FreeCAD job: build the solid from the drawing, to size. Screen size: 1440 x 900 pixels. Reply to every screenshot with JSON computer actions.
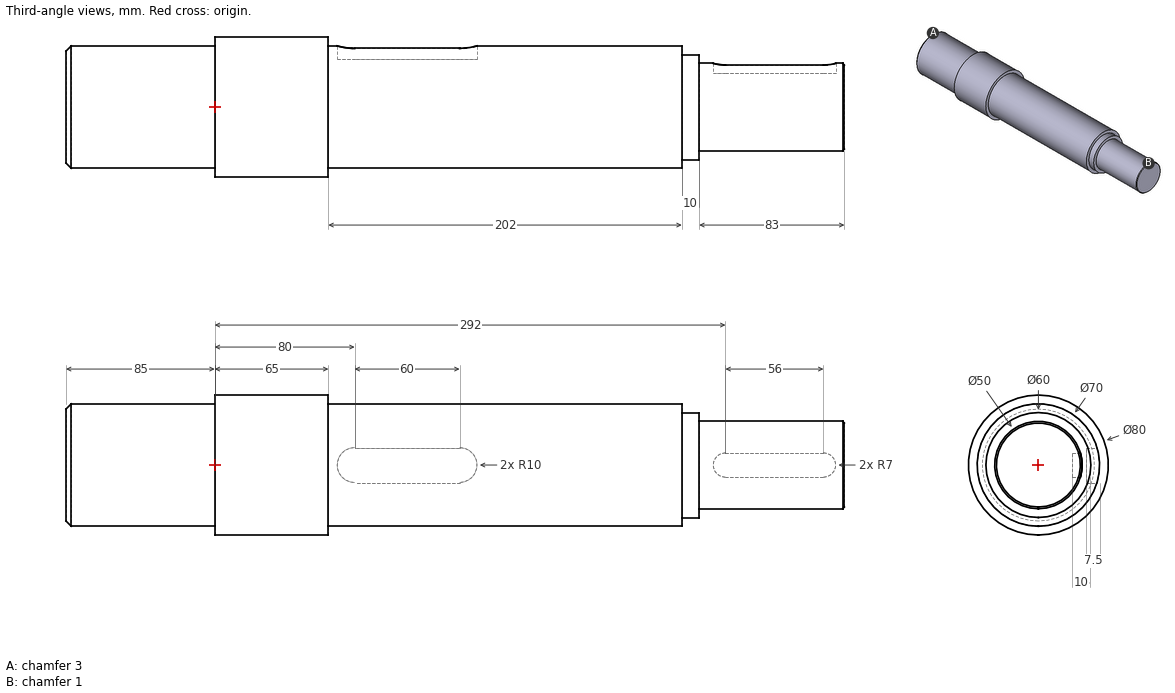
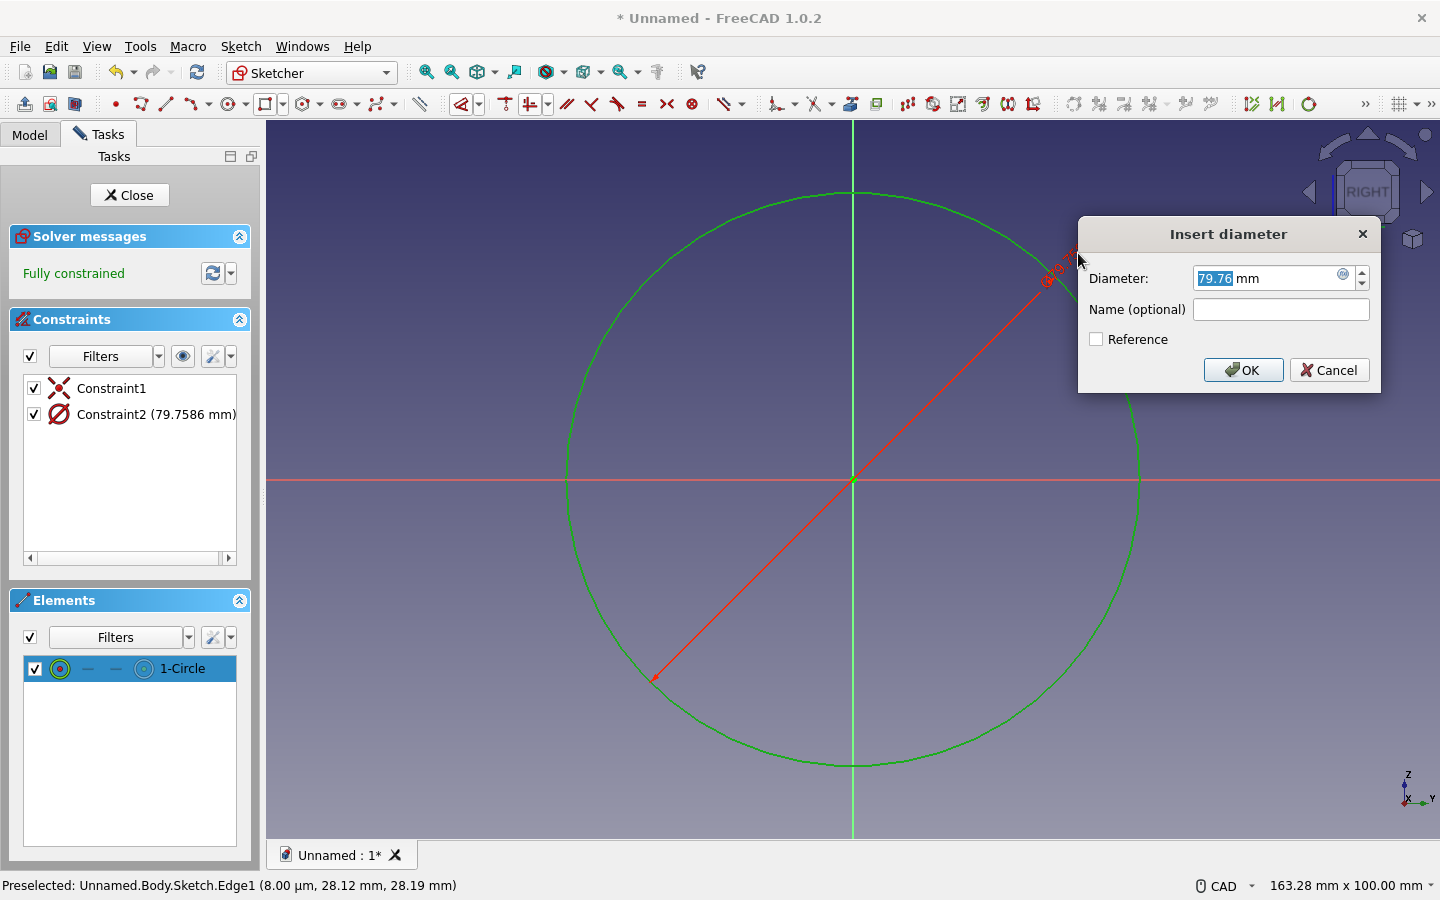
{"action": "type", "text": "80"}
{"action": "key", "text": "Return"}
{"action": "key", "text": "Escape"}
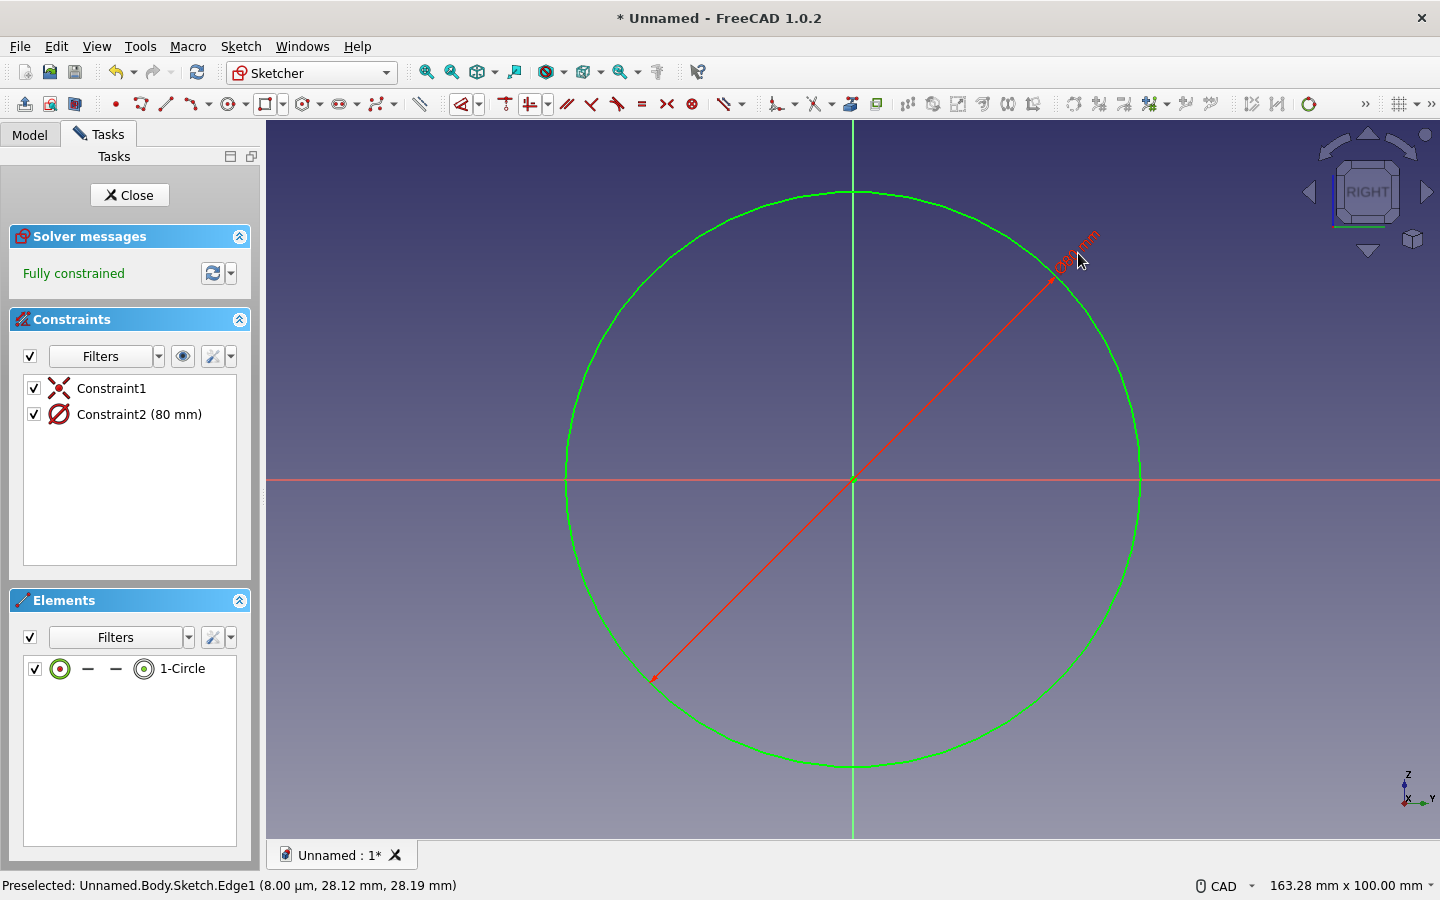
{"action": "left_click", "coordinate": [130, 195]}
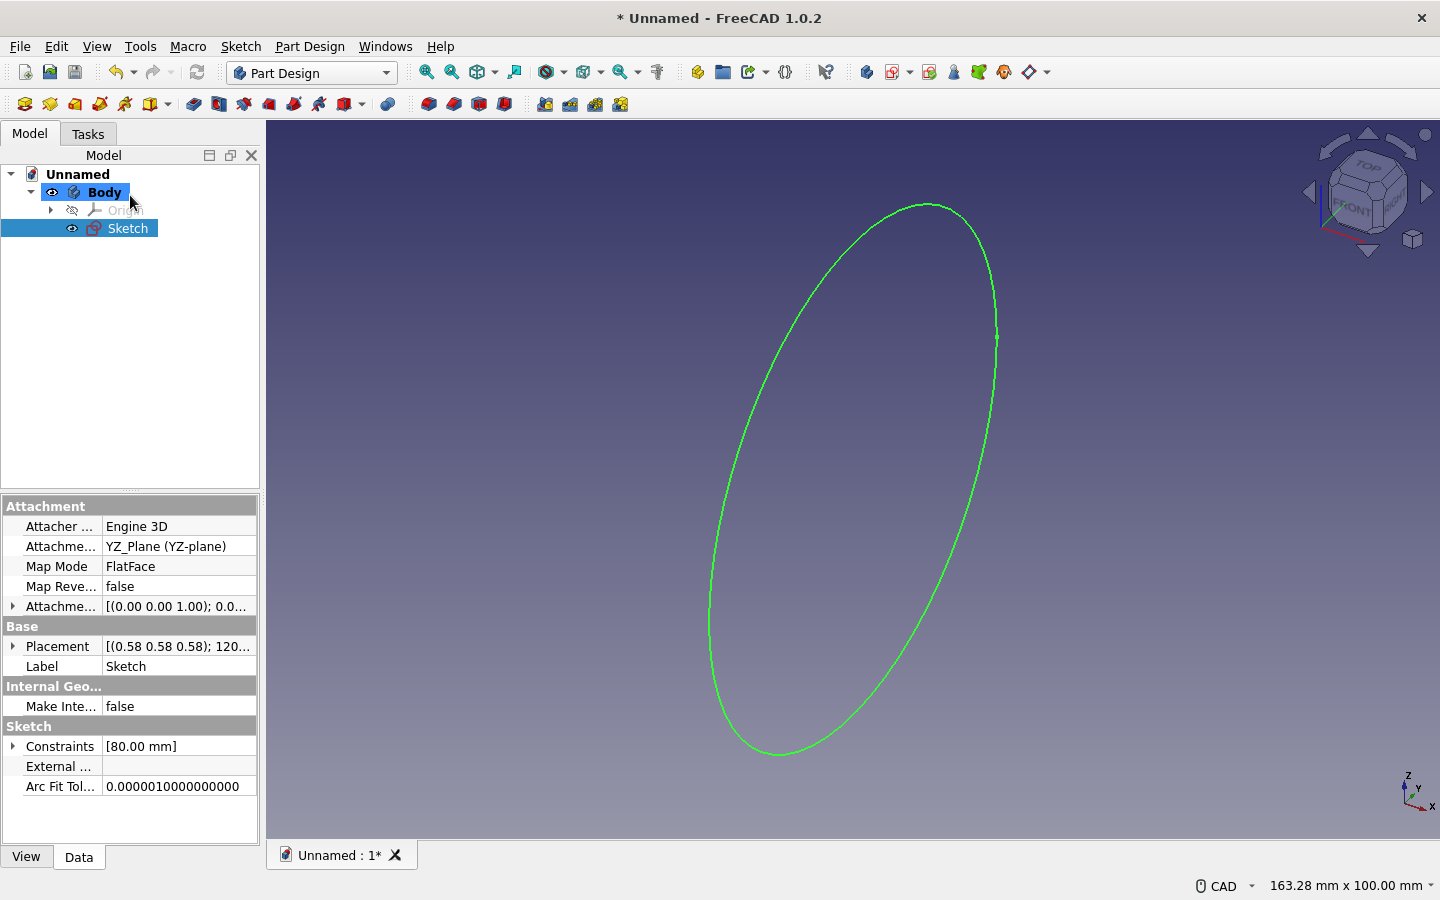
{"action": "left_click", "coordinate": [25, 104]}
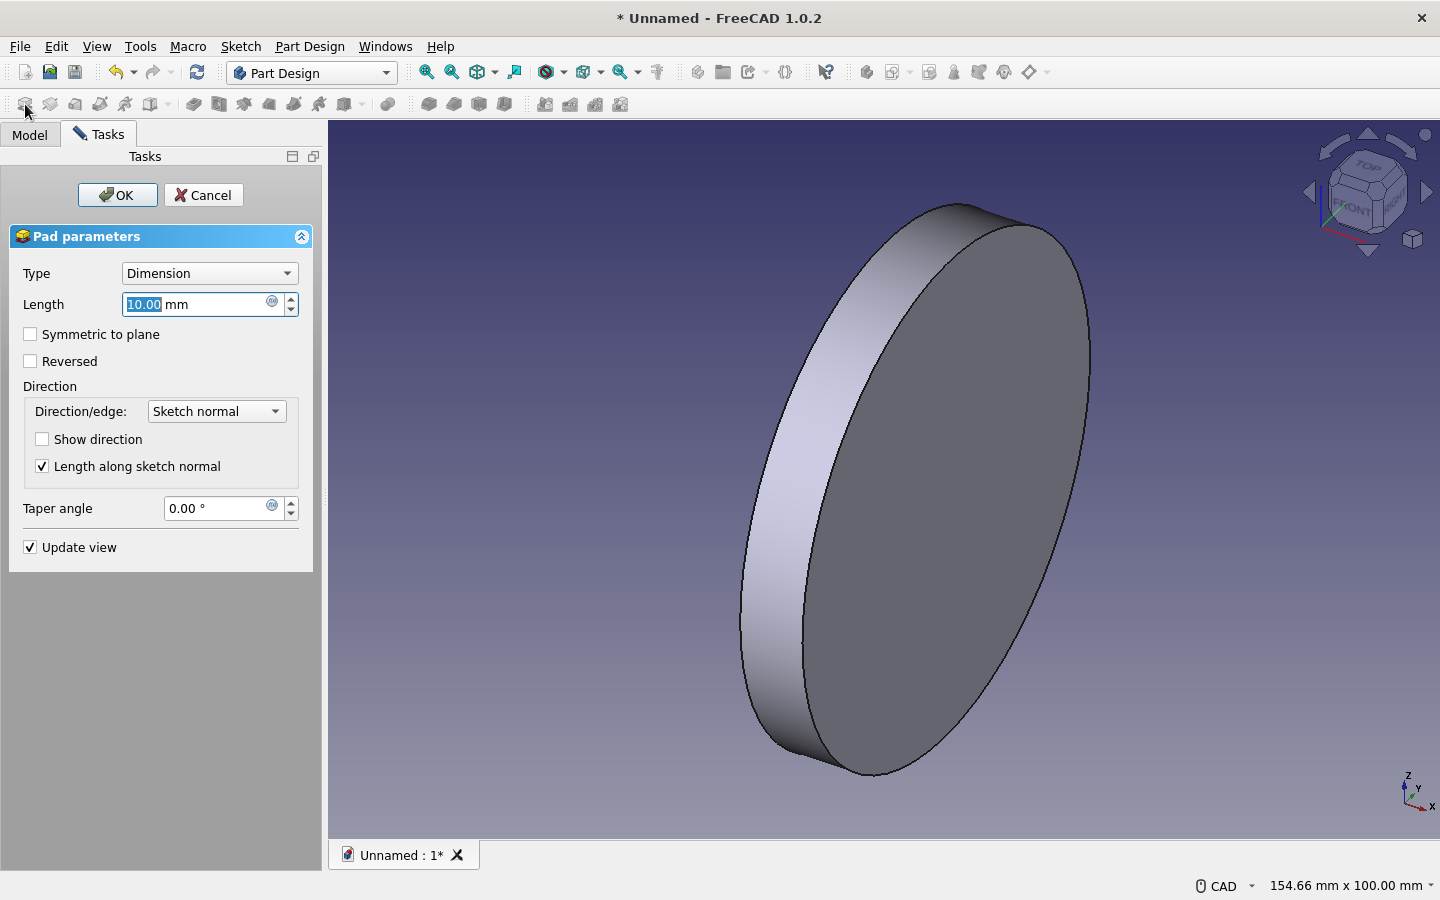
{"action": "type", "text": "65"}
{"action": "key", "text": "Tab"}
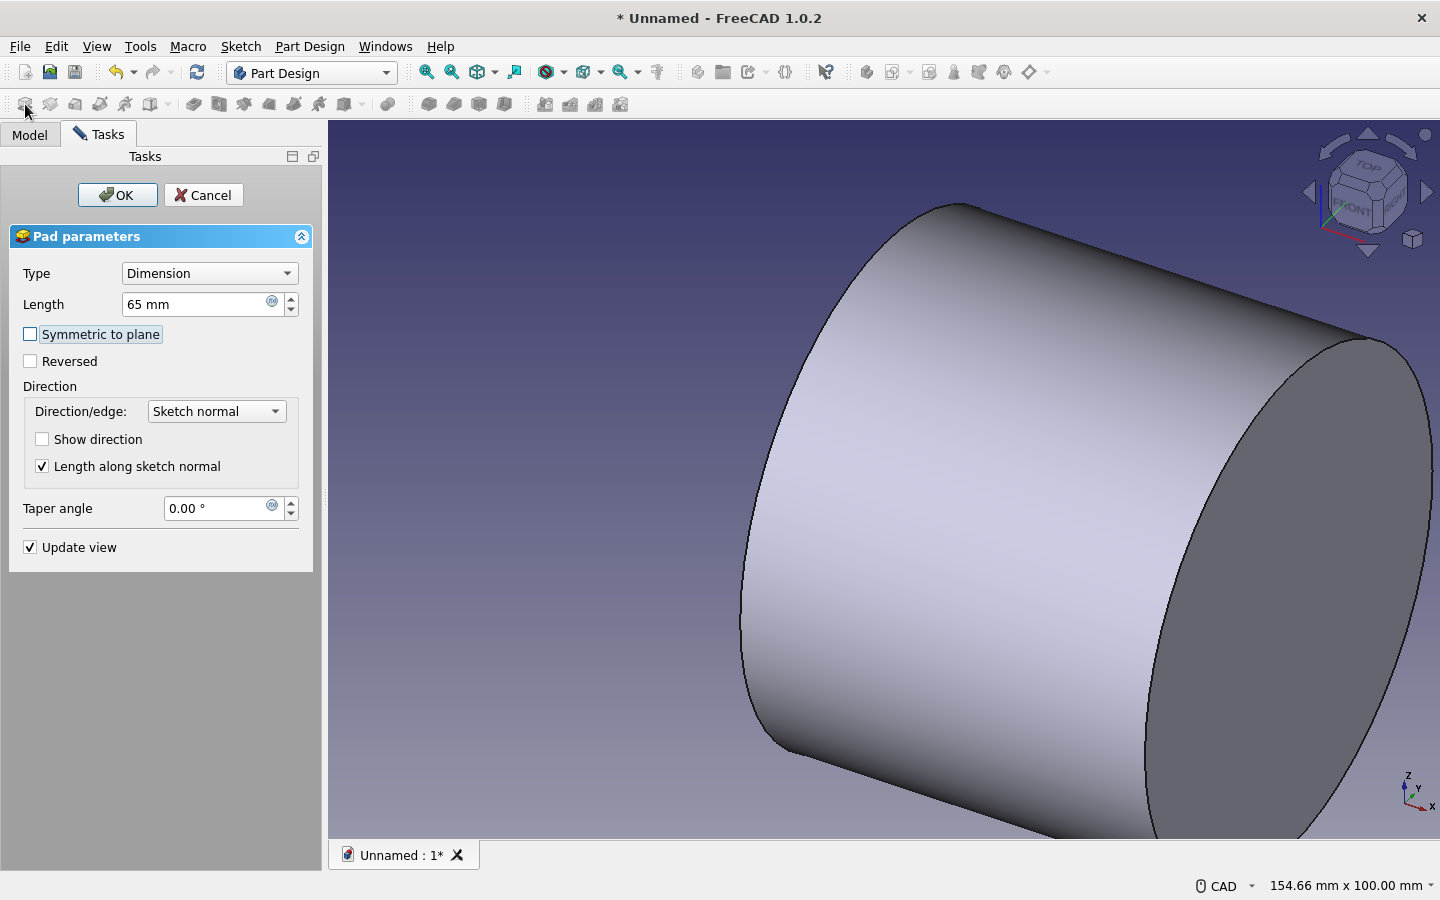
{"action": "left_click", "coordinate": [118, 195]}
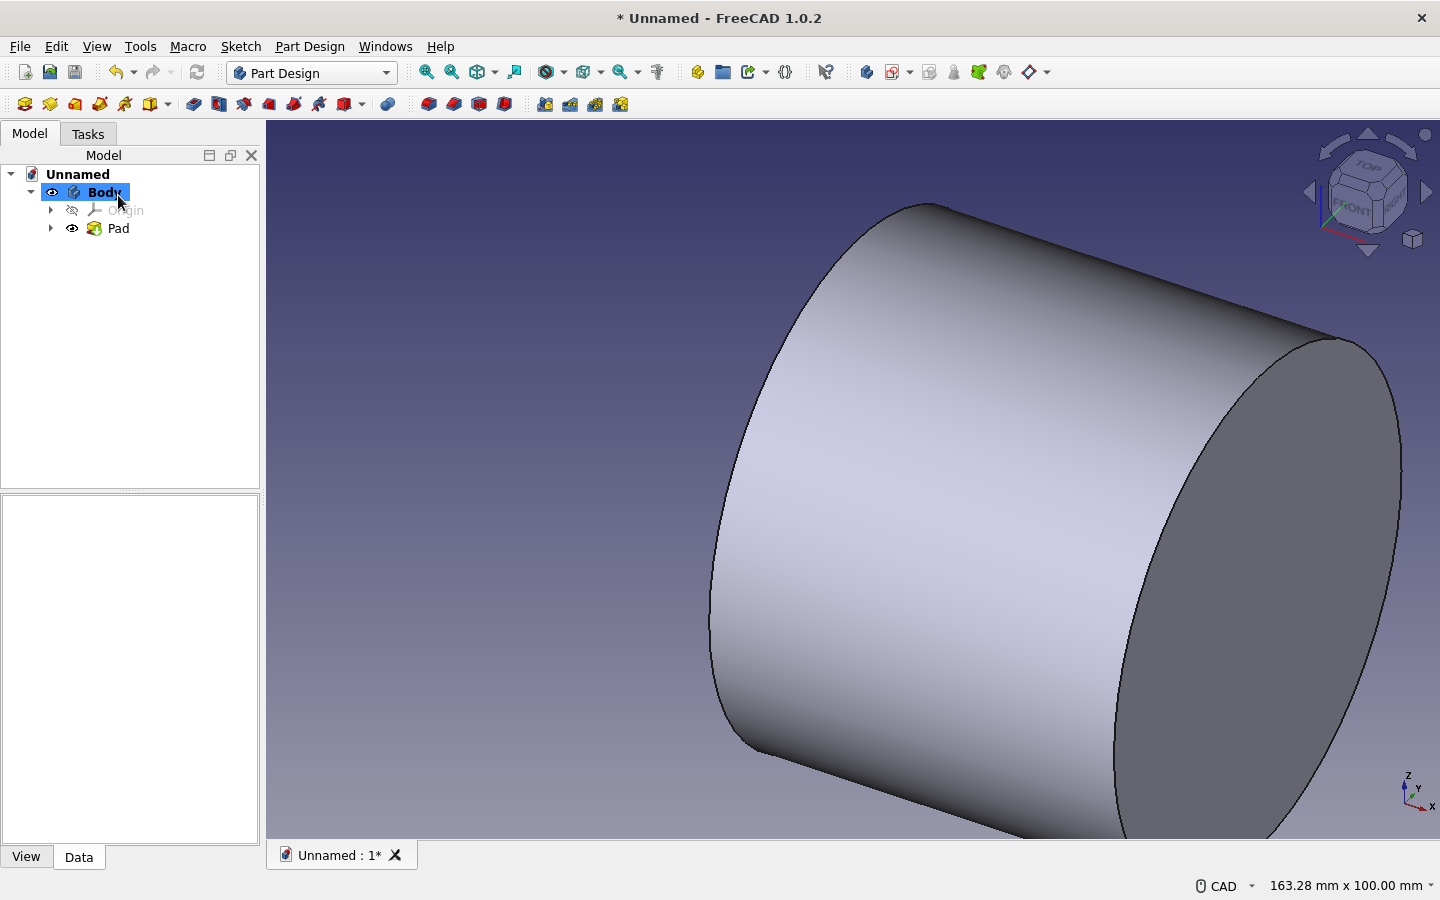
{"action": "key", "text": "v f"}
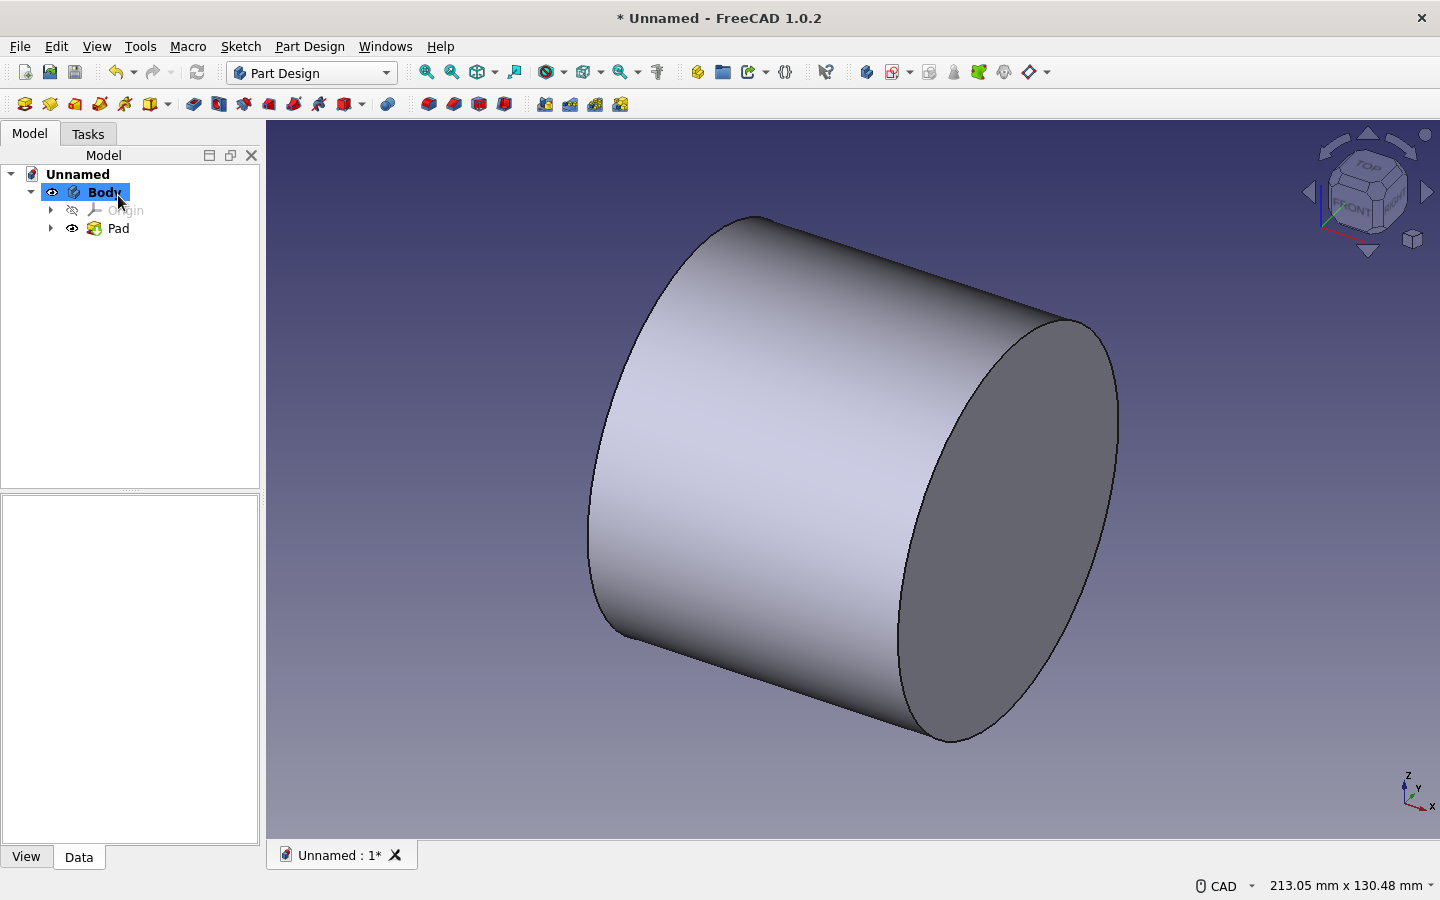
{"action": "left_click", "coordinate": [1008, 530]}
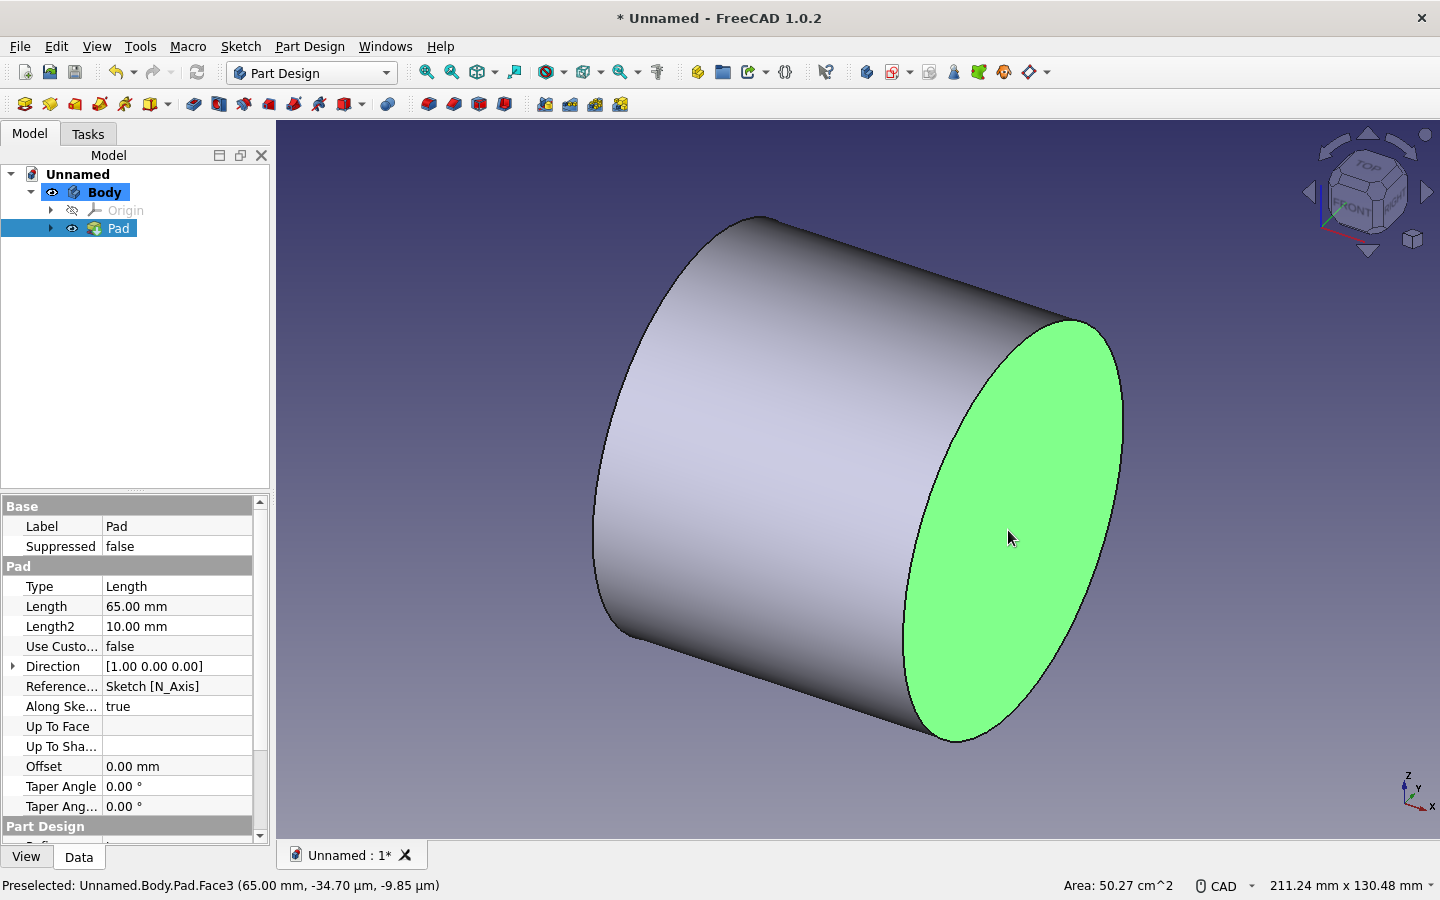
{"action": "left_click", "coordinate": [892, 72]}